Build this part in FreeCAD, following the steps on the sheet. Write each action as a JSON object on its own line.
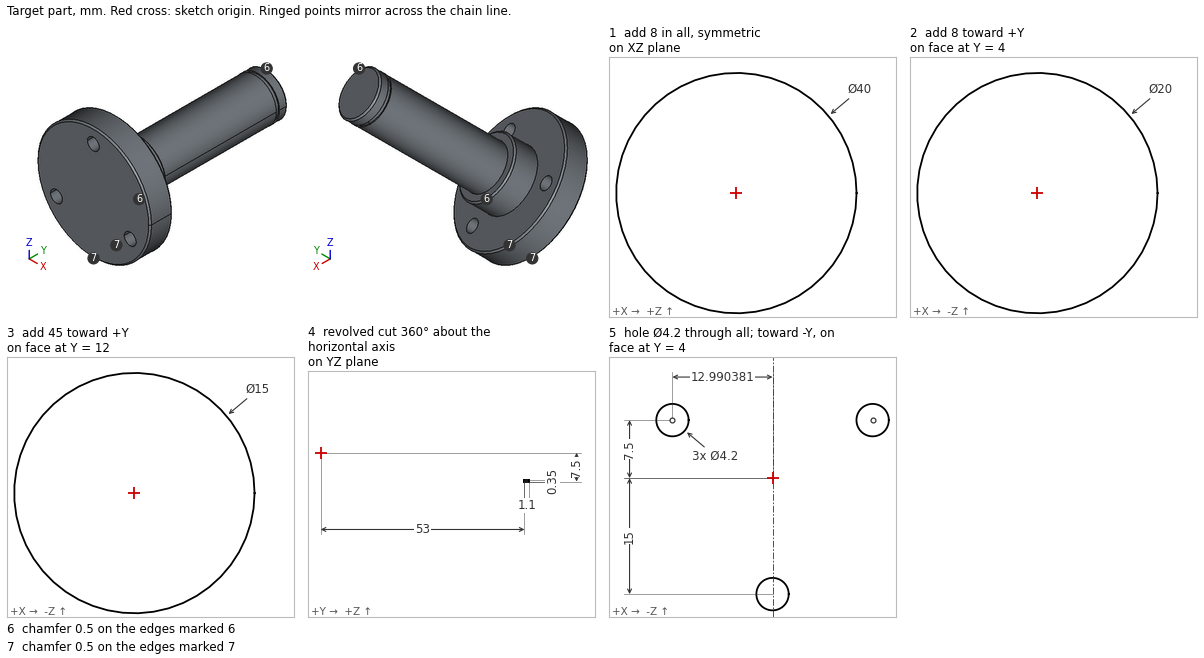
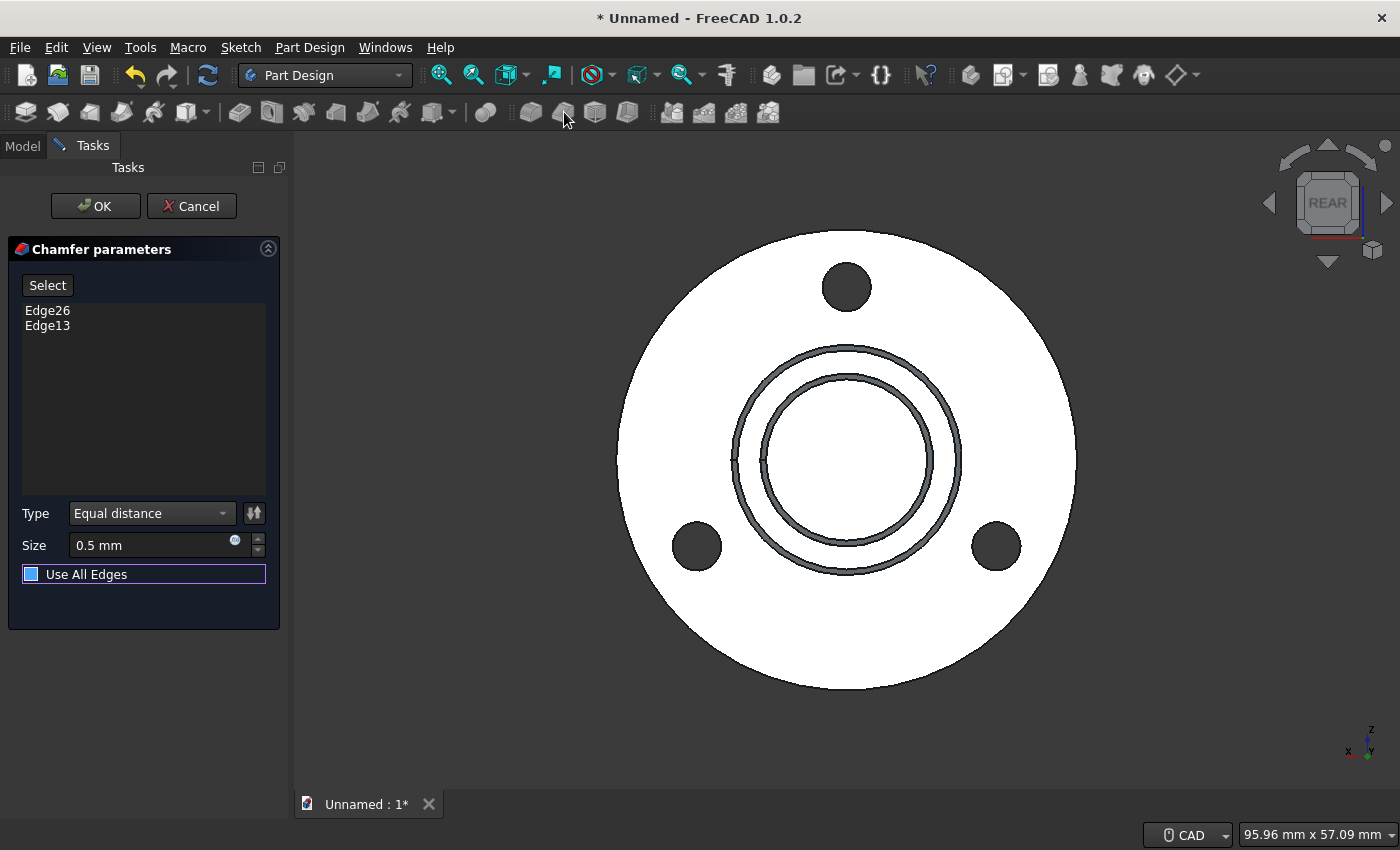
{"action": "left_click", "coordinate": [96, 206]}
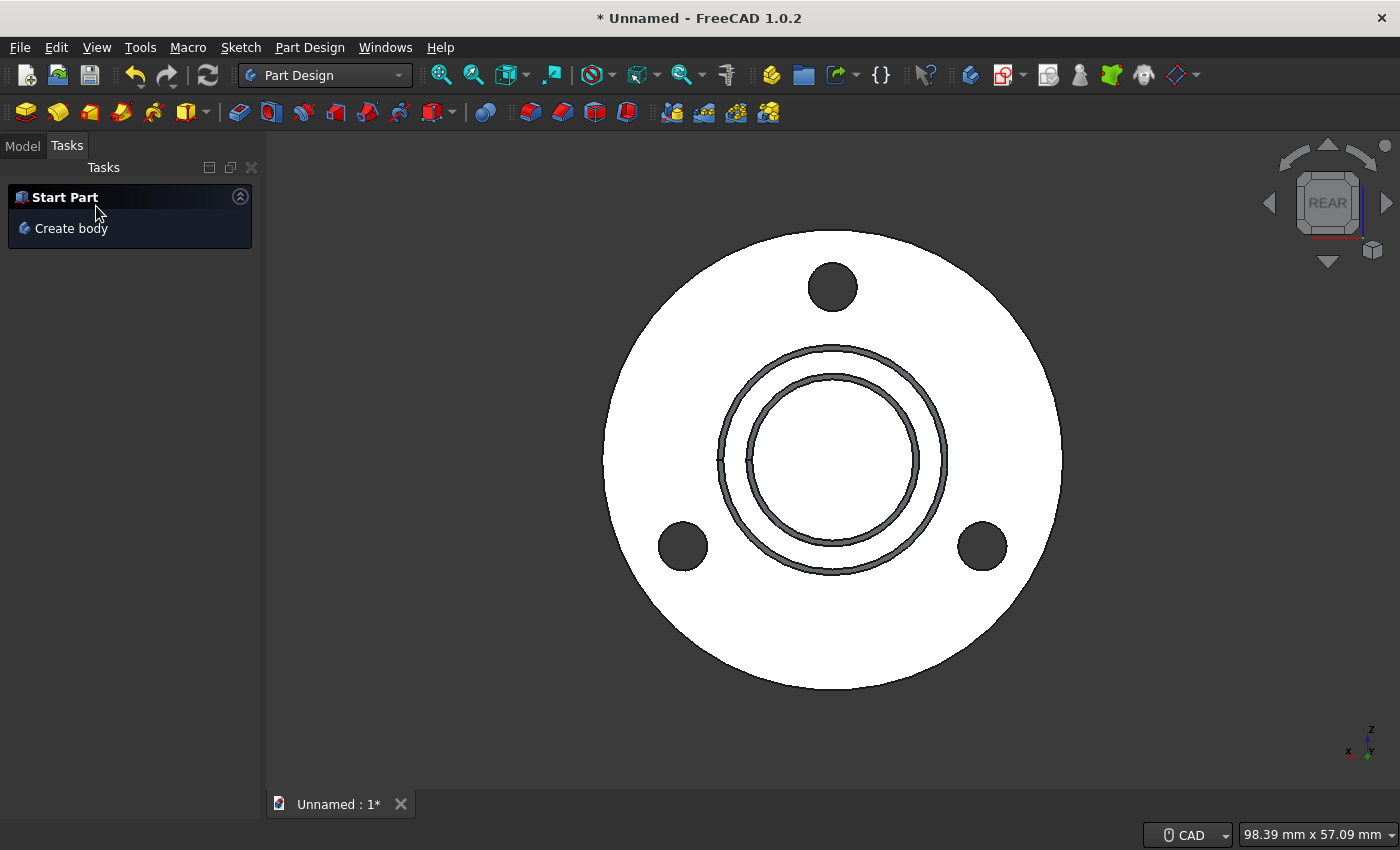
{"action": "left_click", "coordinate": [1063, 459]}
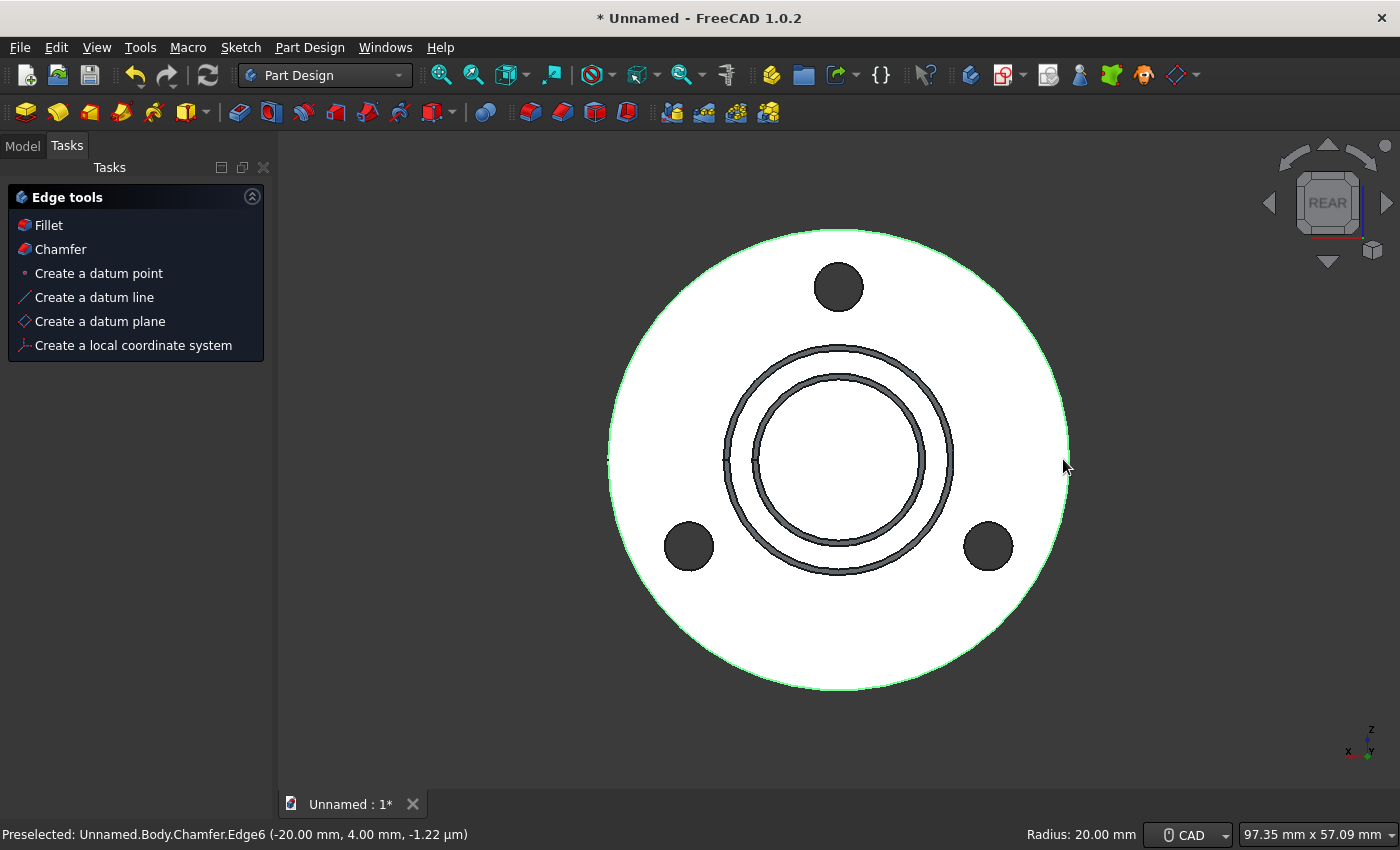
{"action": "key", "text": "0"}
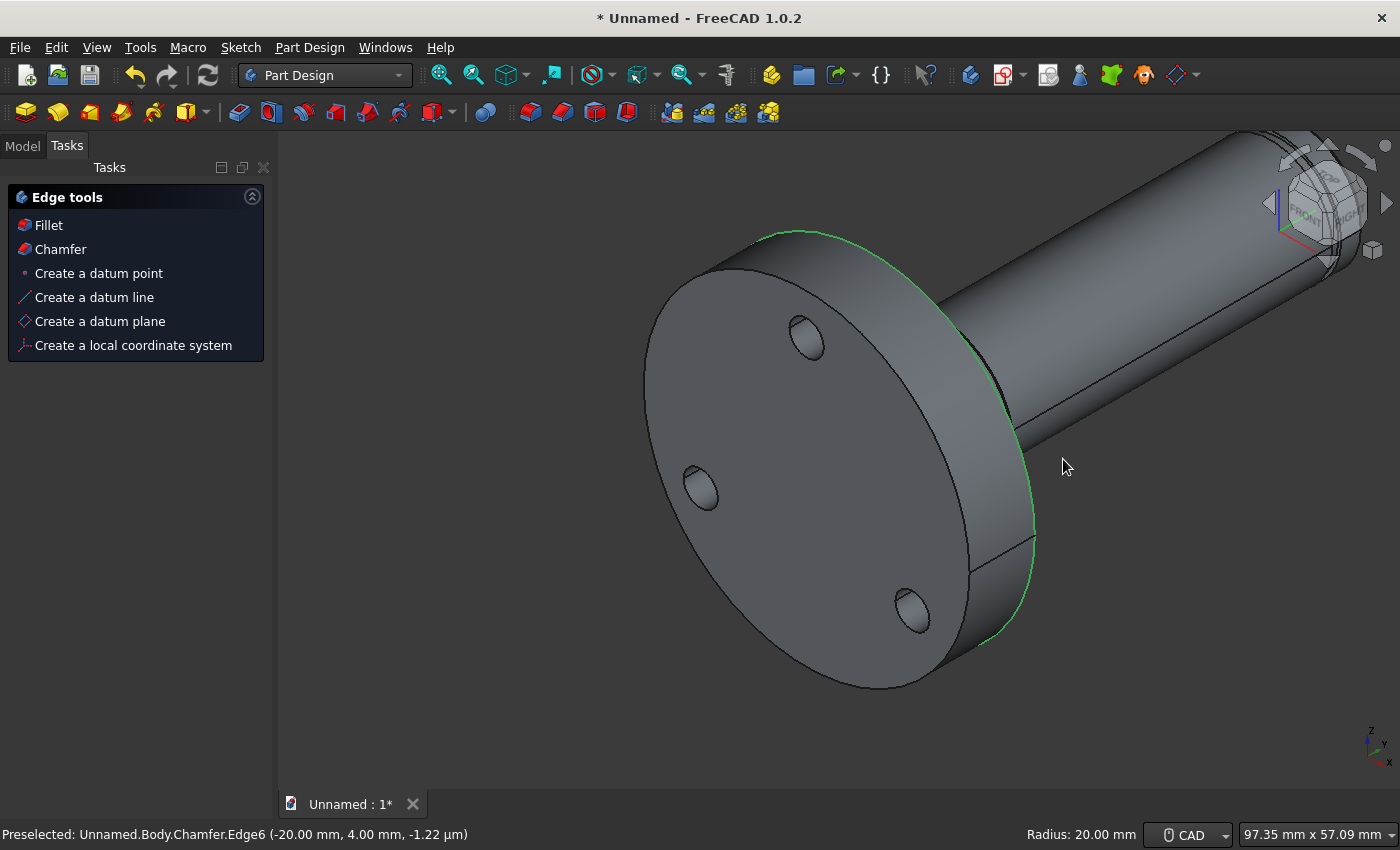
{"action": "left_click", "coordinate": [442, 76]}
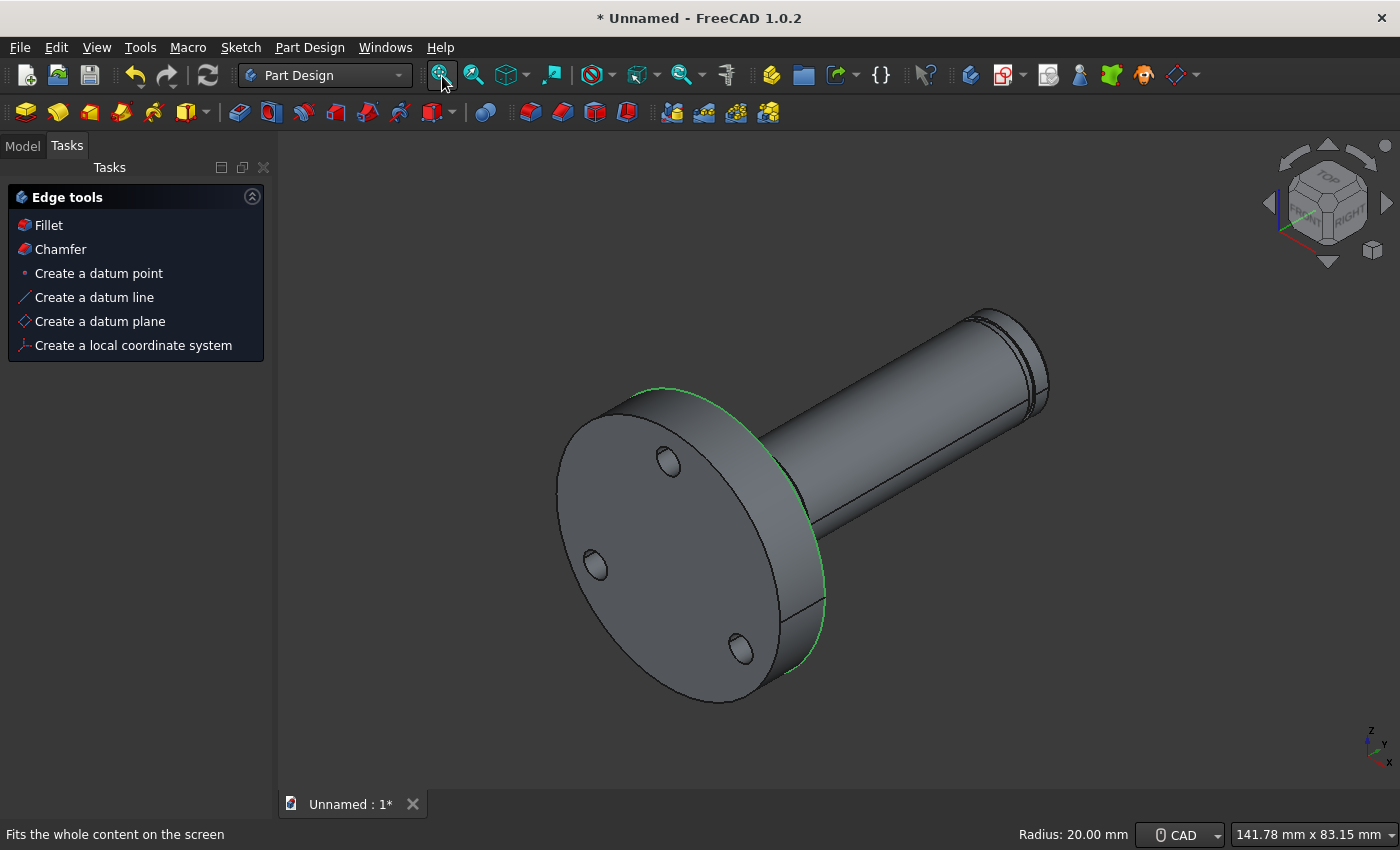
{"action": "left_click", "coordinate": [634, 415], "text": "ctrl"}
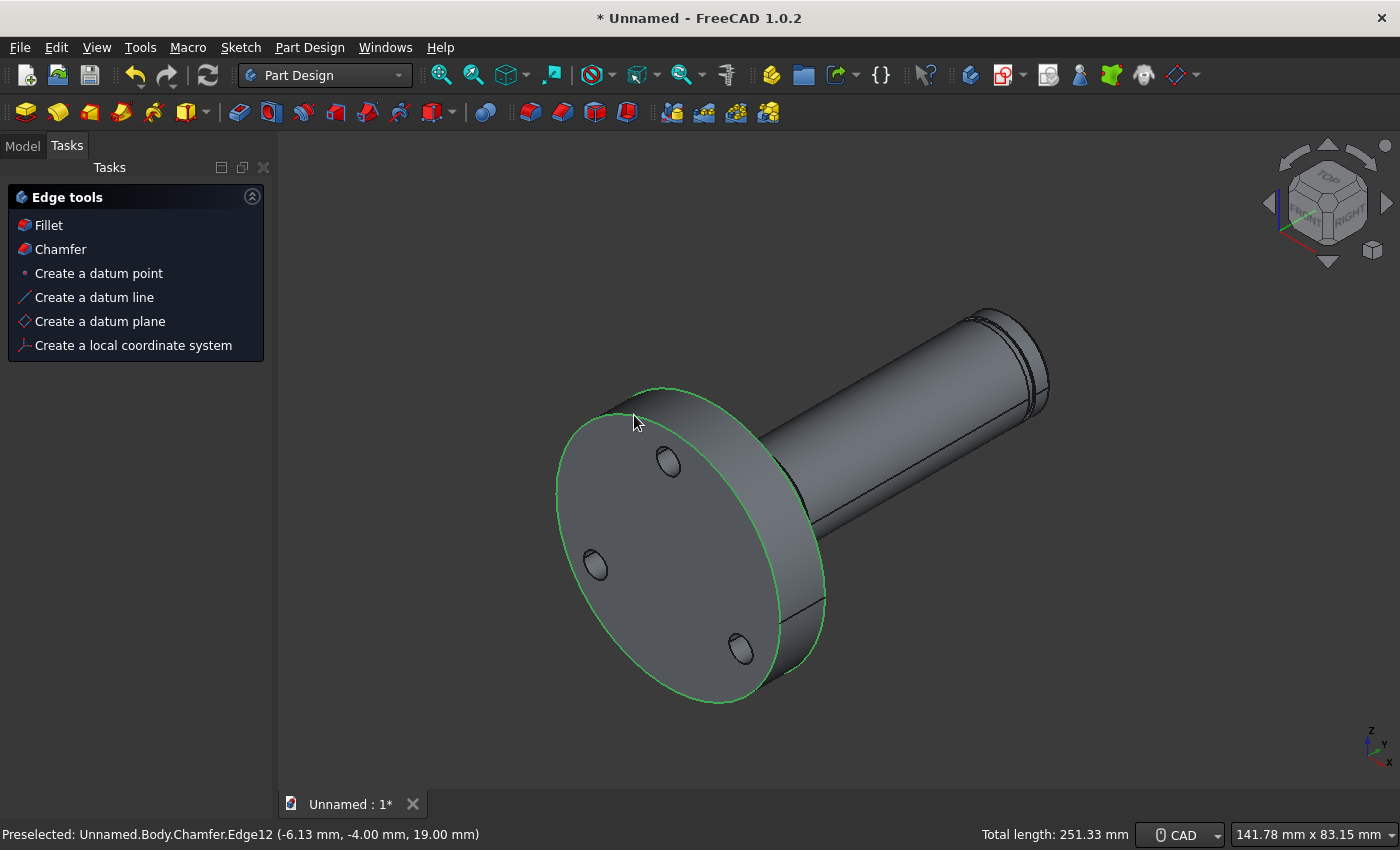
{"action": "left_click", "coordinate": [564, 112]}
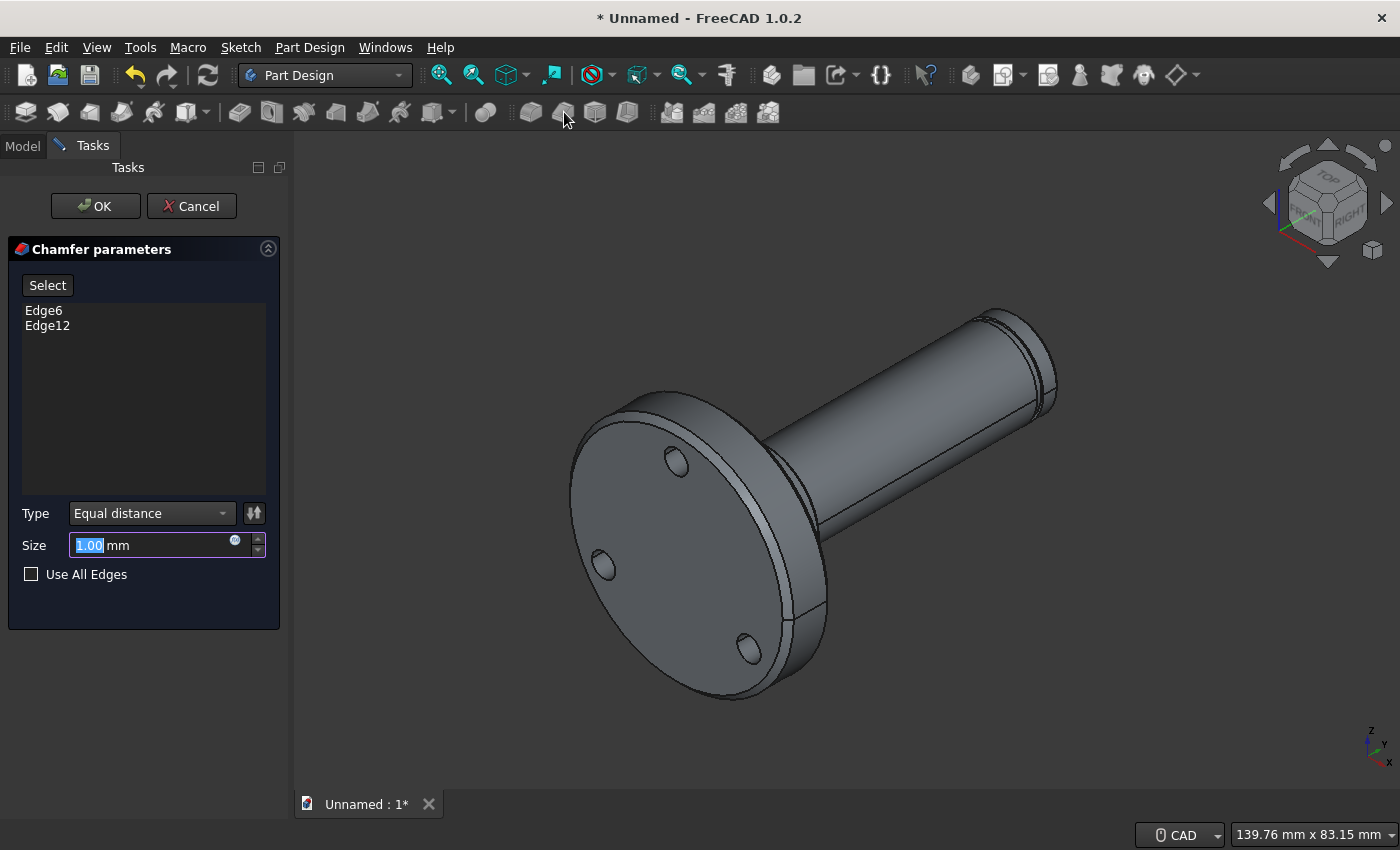
{"action": "type", "text": "0.5"}
{"action": "key", "text": "Tab"}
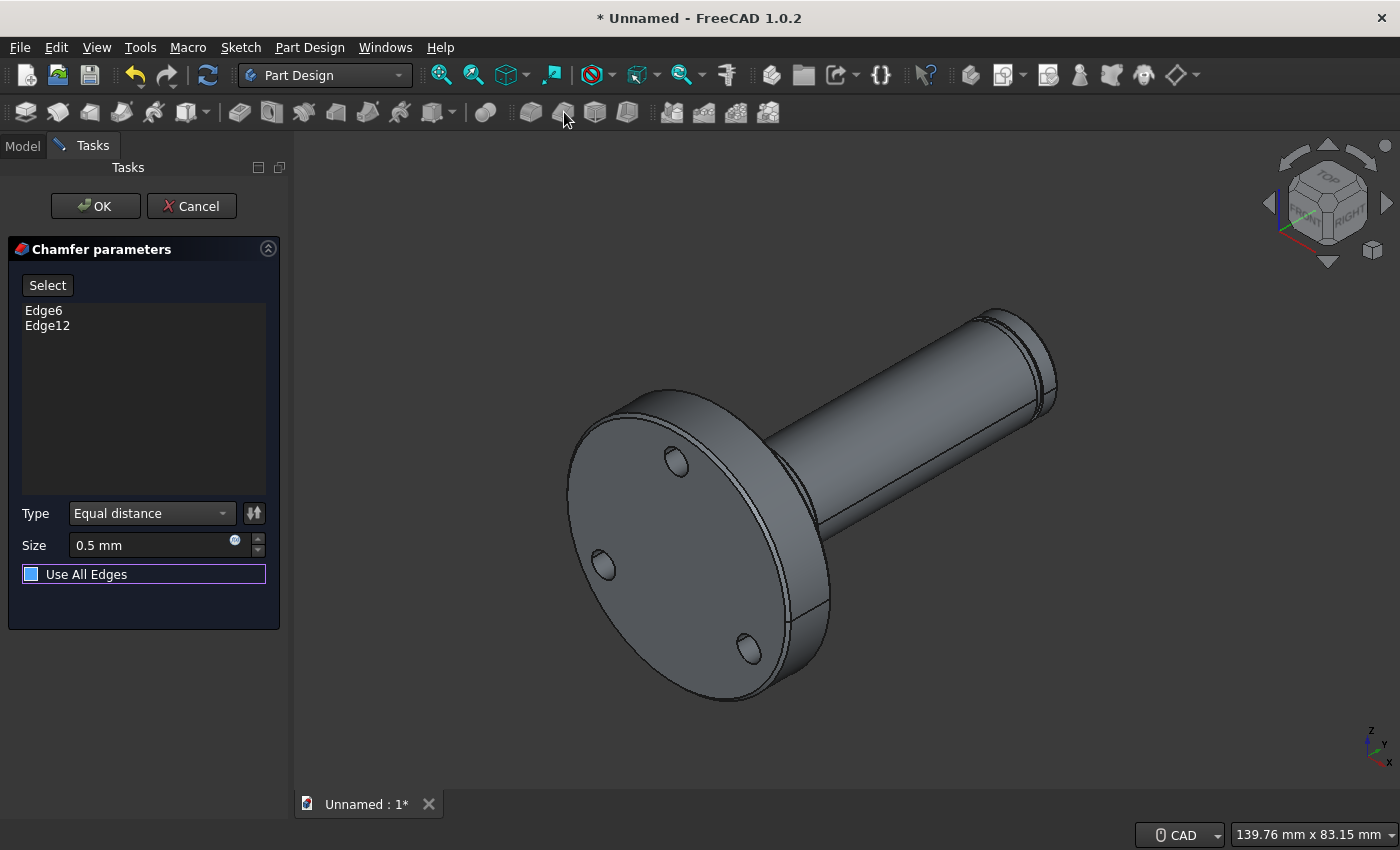
{"action": "left_click", "coordinate": [96, 206]}